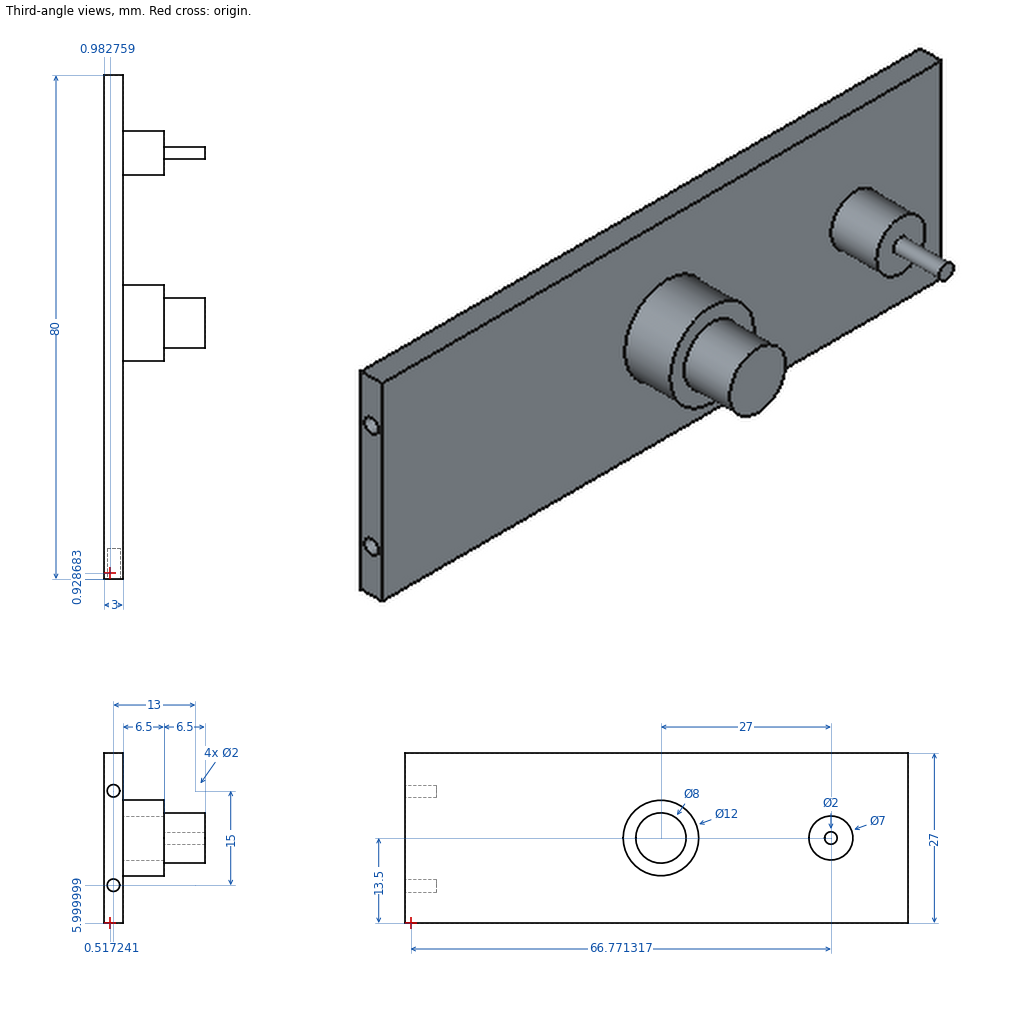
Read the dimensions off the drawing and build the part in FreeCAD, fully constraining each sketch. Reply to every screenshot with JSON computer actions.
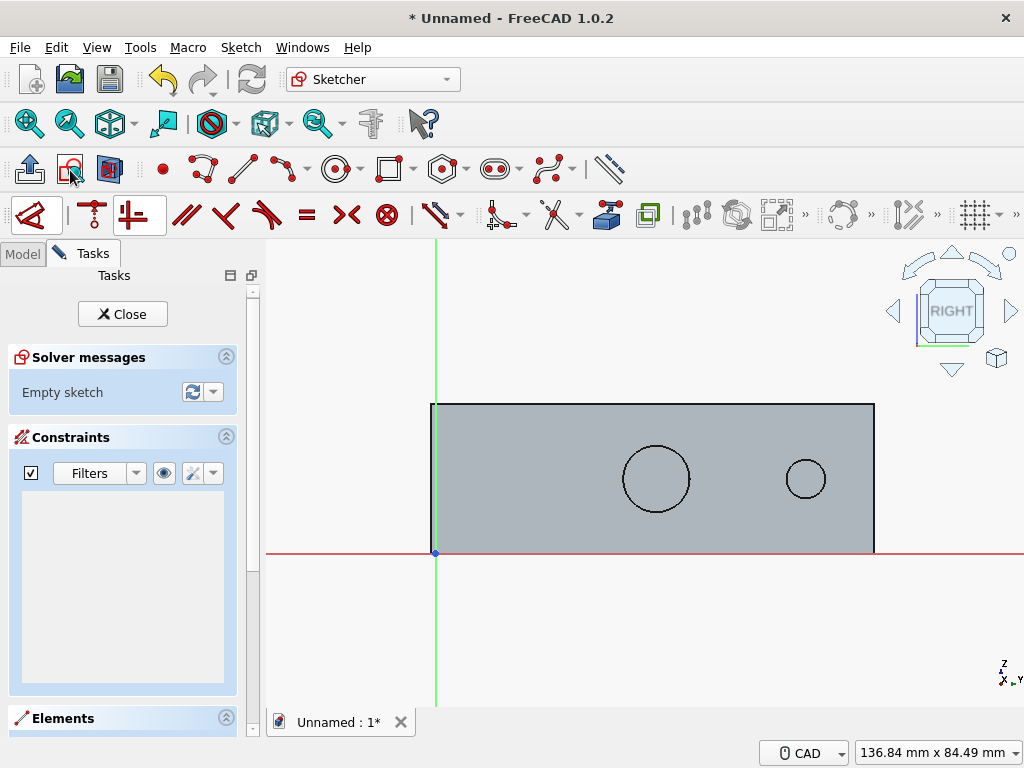
{"action": "left_click", "coordinate": [336, 170]}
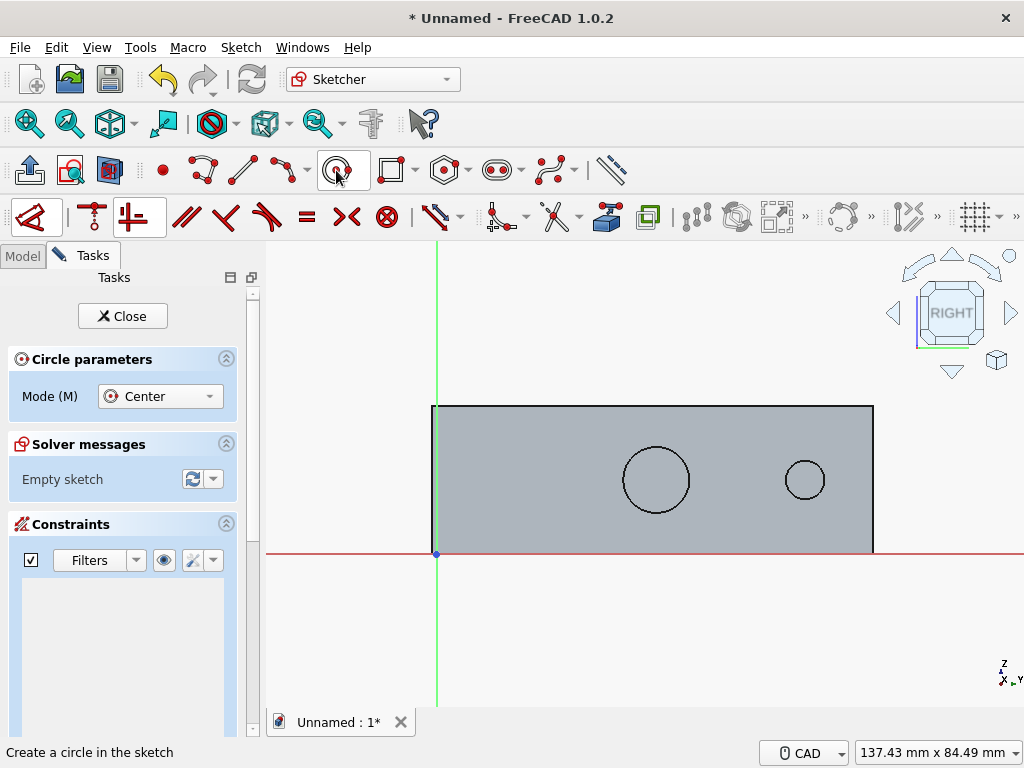
{"action": "scroll", "coordinate": [805, 480], "scroll_direction": "up", "scroll_amount": 8}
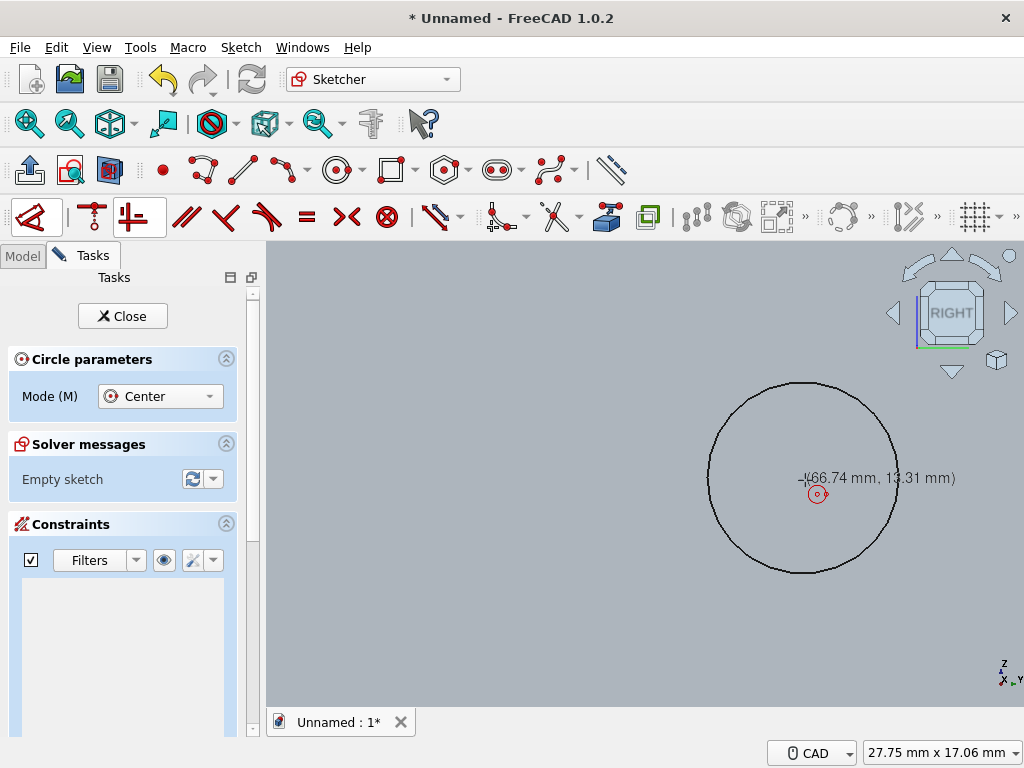
{"action": "scroll", "coordinate": [746, 440], "scroll_direction": "down", "scroll_amount": 8}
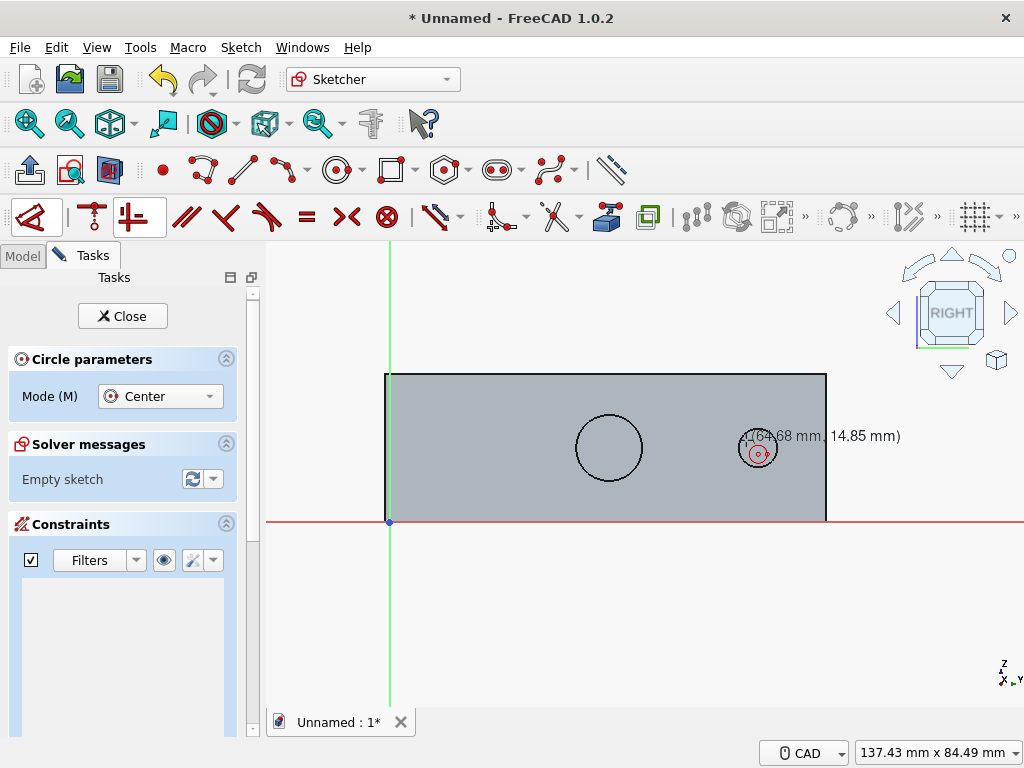
{"action": "left_click", "coordinate": [758, 448]}
{"action": "mouse_move", "coordinate": [762, 444]}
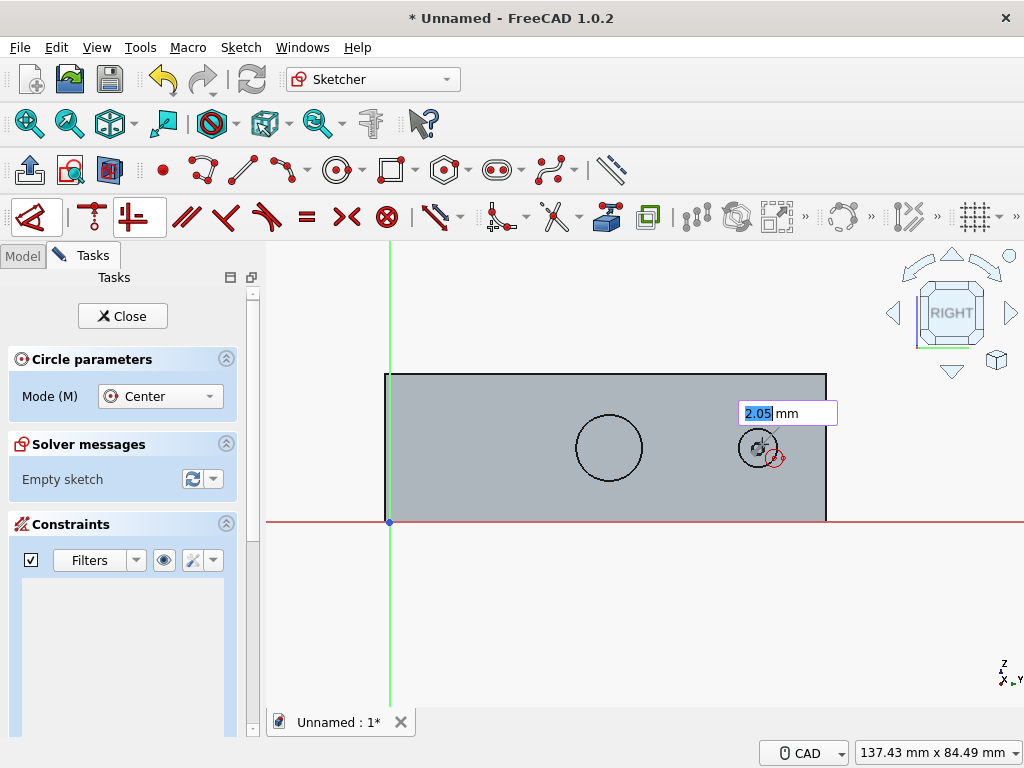
{"action": "type", "text": "2"}
{"action": "key", "text": "Return"}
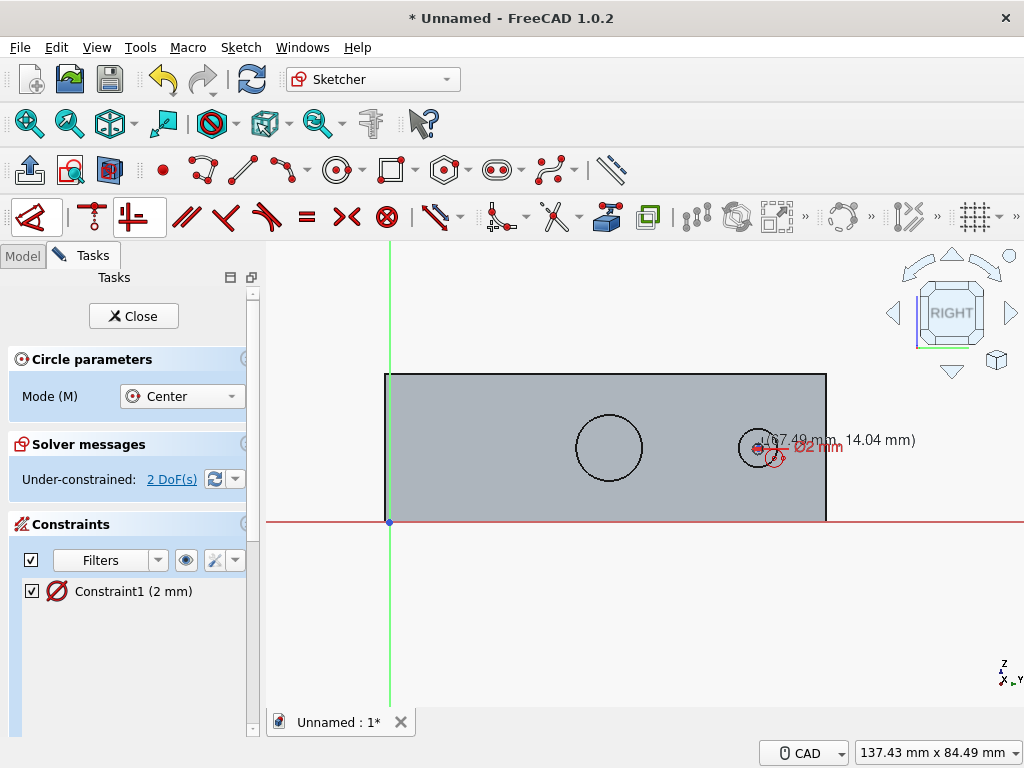
{"action": "left_click", "coordinate": [609, 448]}
{"action": "mouse_move", "coordinate": [625, 432]}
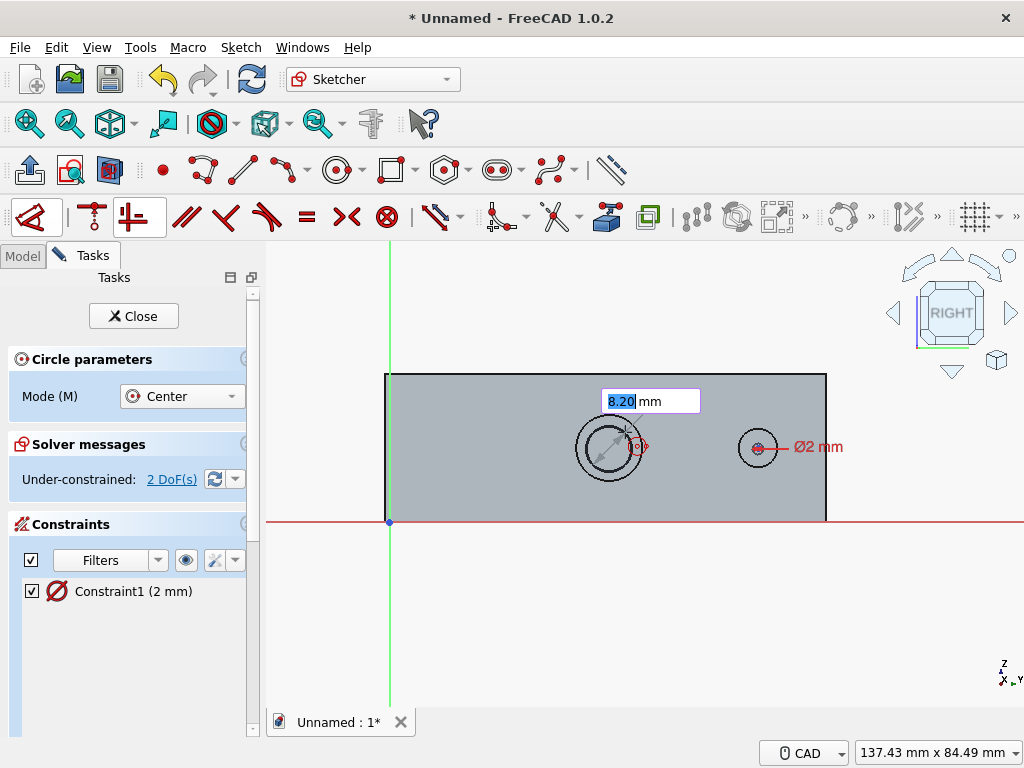
{"action": "type", "text": "8"}
{"action": "key", "text": "Return"}
{"action": "key", "text": "Escape"}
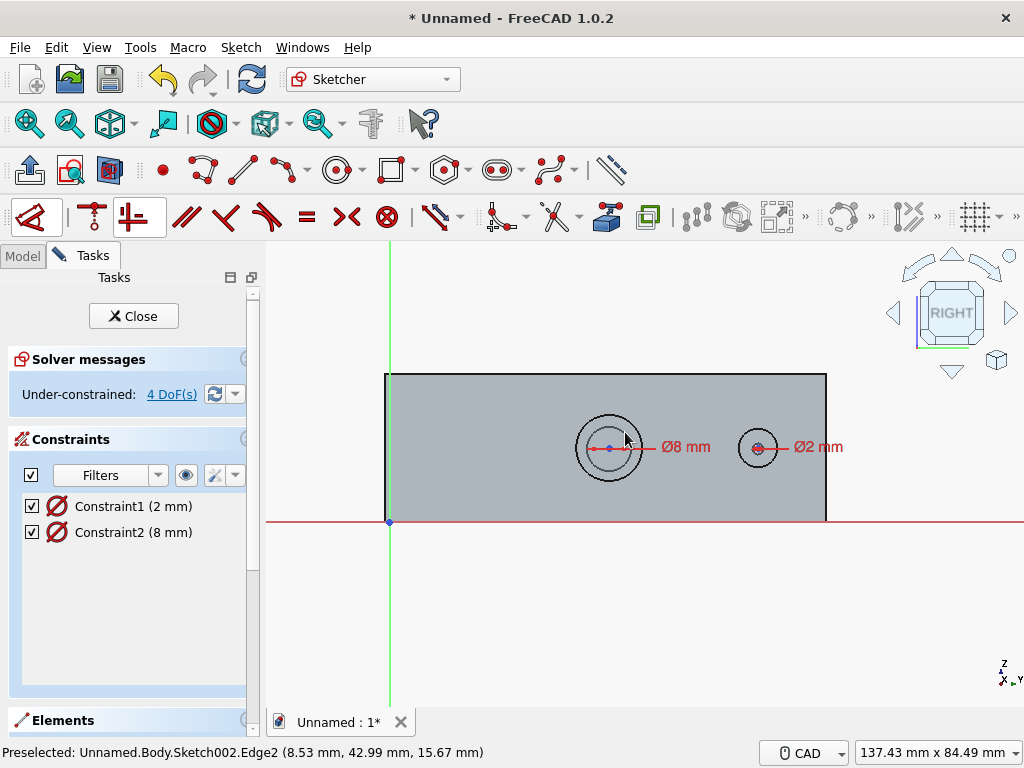
{"action": "left_click", "coordinate": [758, 449]}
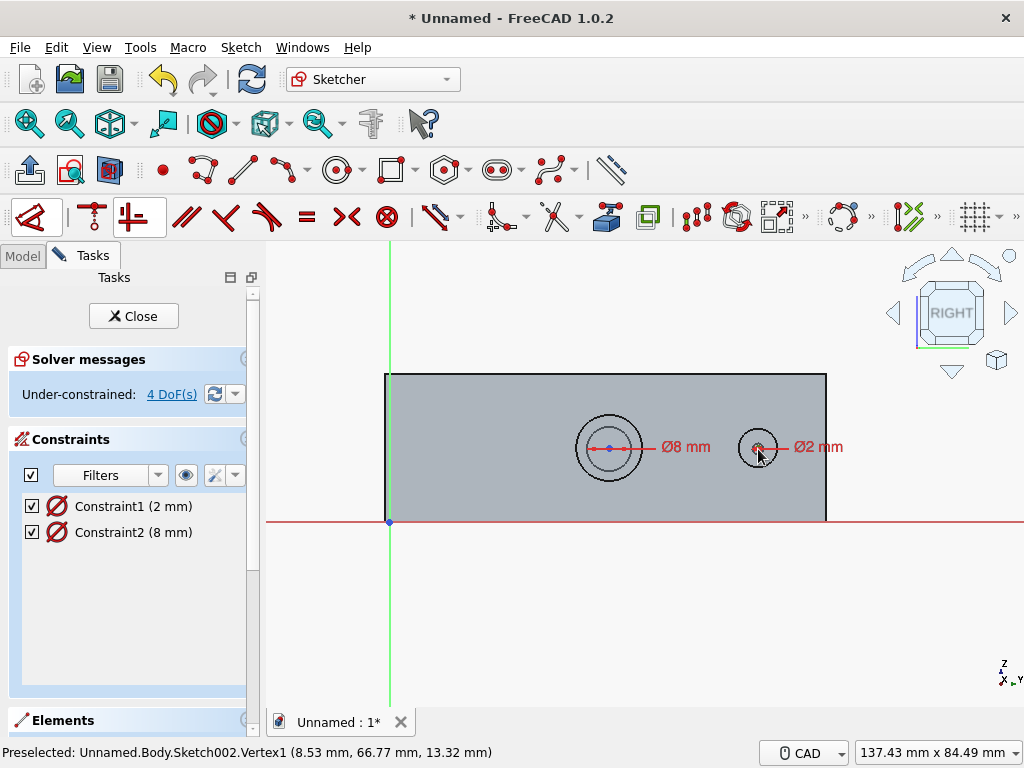
{"action": "left_click", "coordinate": [609, 449]}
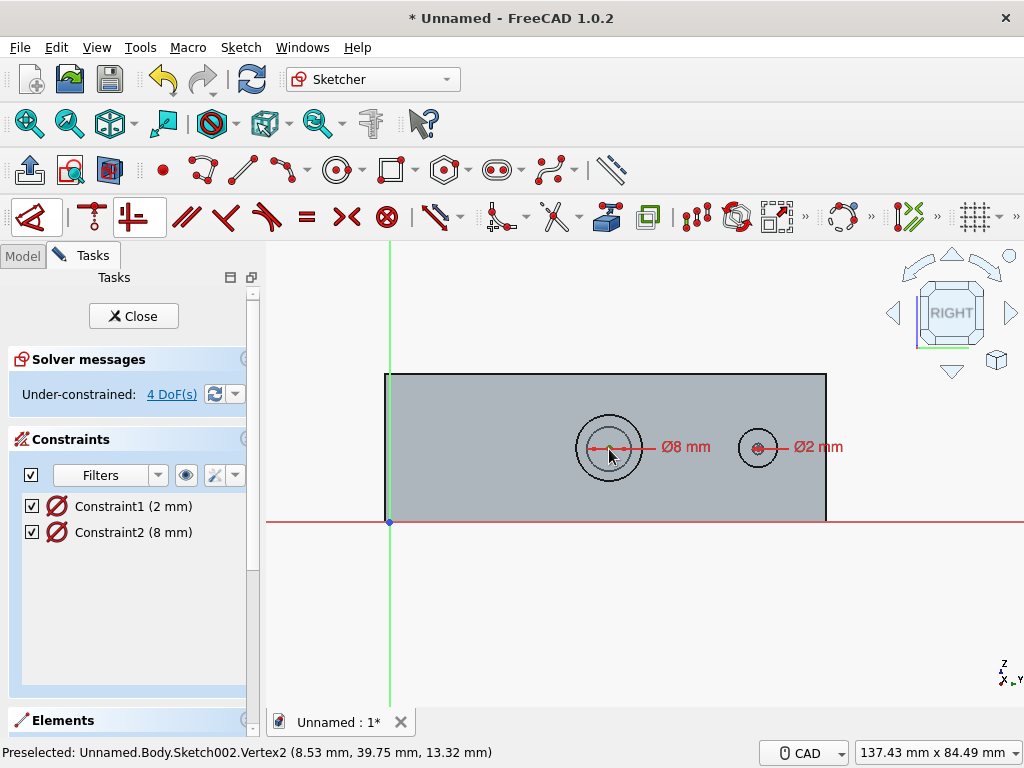
{"action": "left_click", "coordinate": [160, 218]}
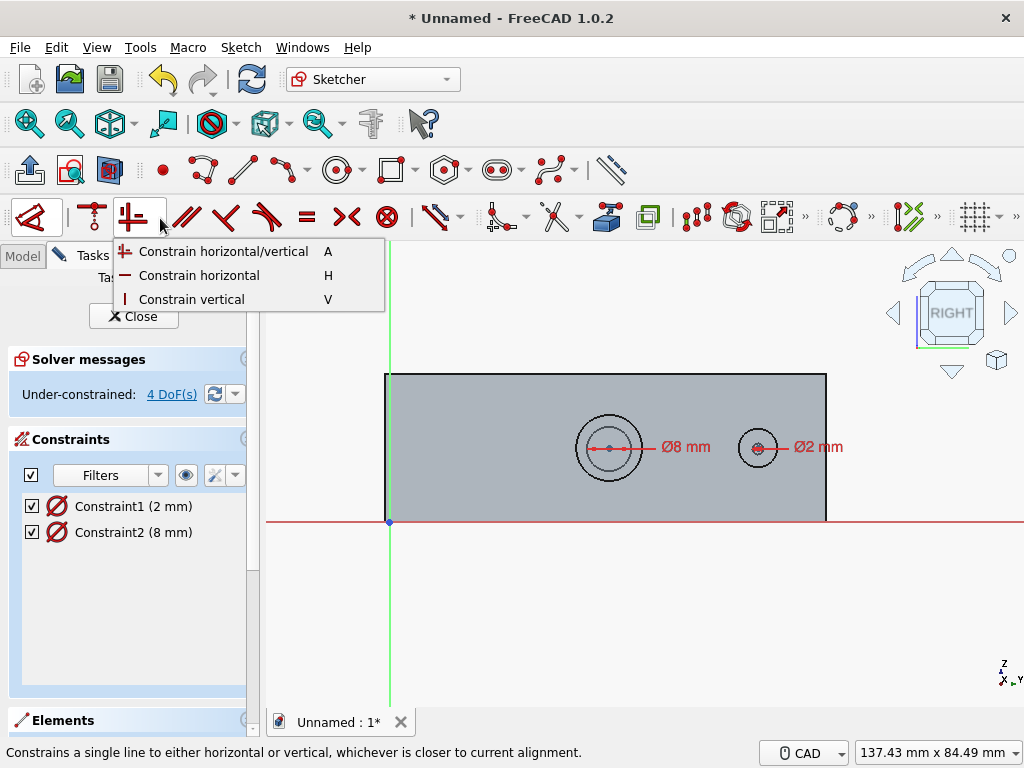
{"action": "left_click", "coordinate": [249, 275]}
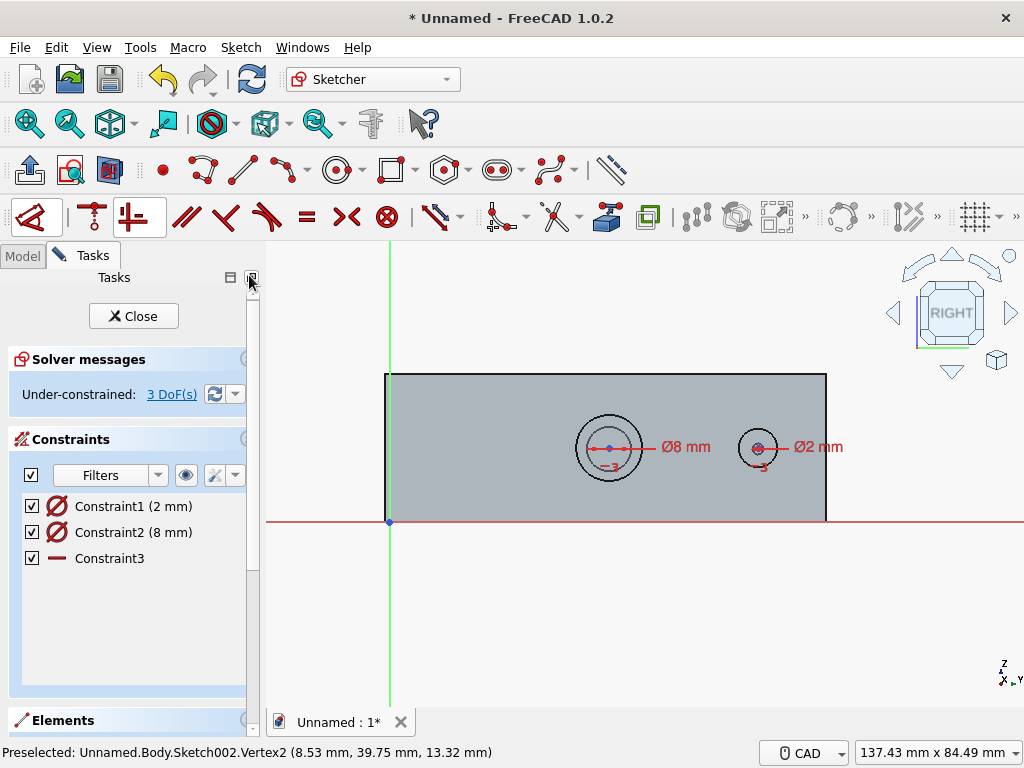
{"action": "left_click", "coordinate": [758, 449]}